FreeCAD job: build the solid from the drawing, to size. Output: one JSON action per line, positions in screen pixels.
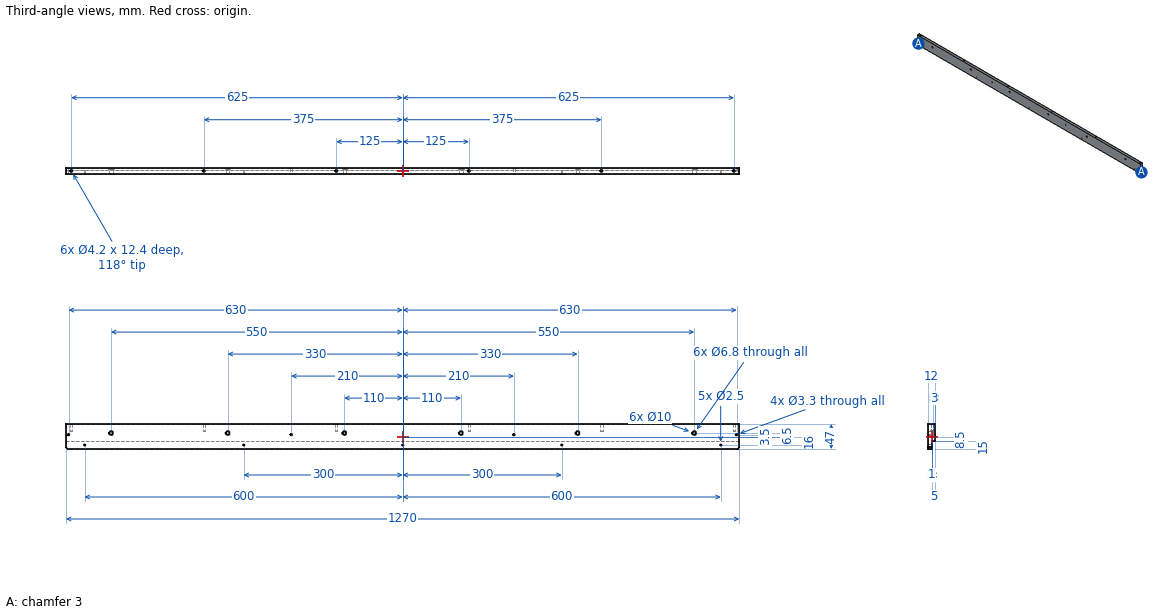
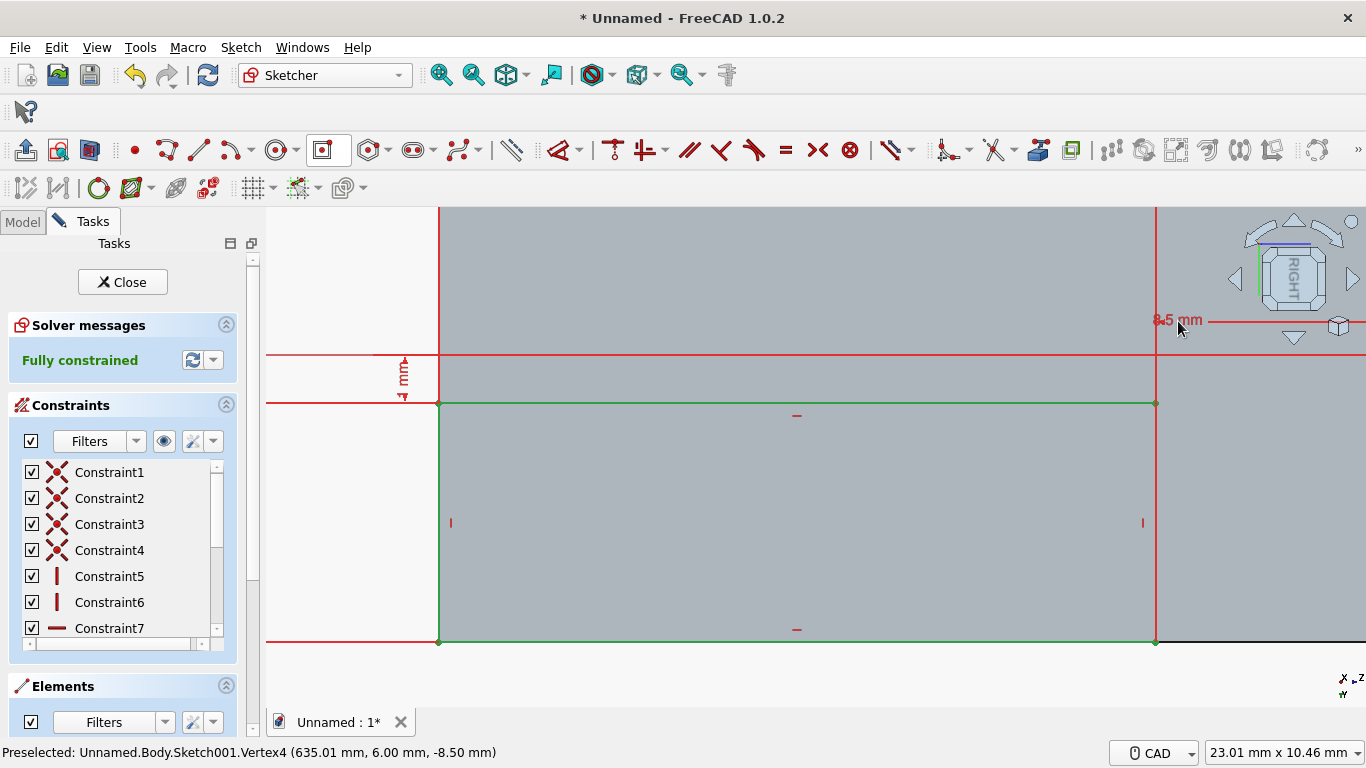
{"action": "left_click", "coordinate": [123, 282]}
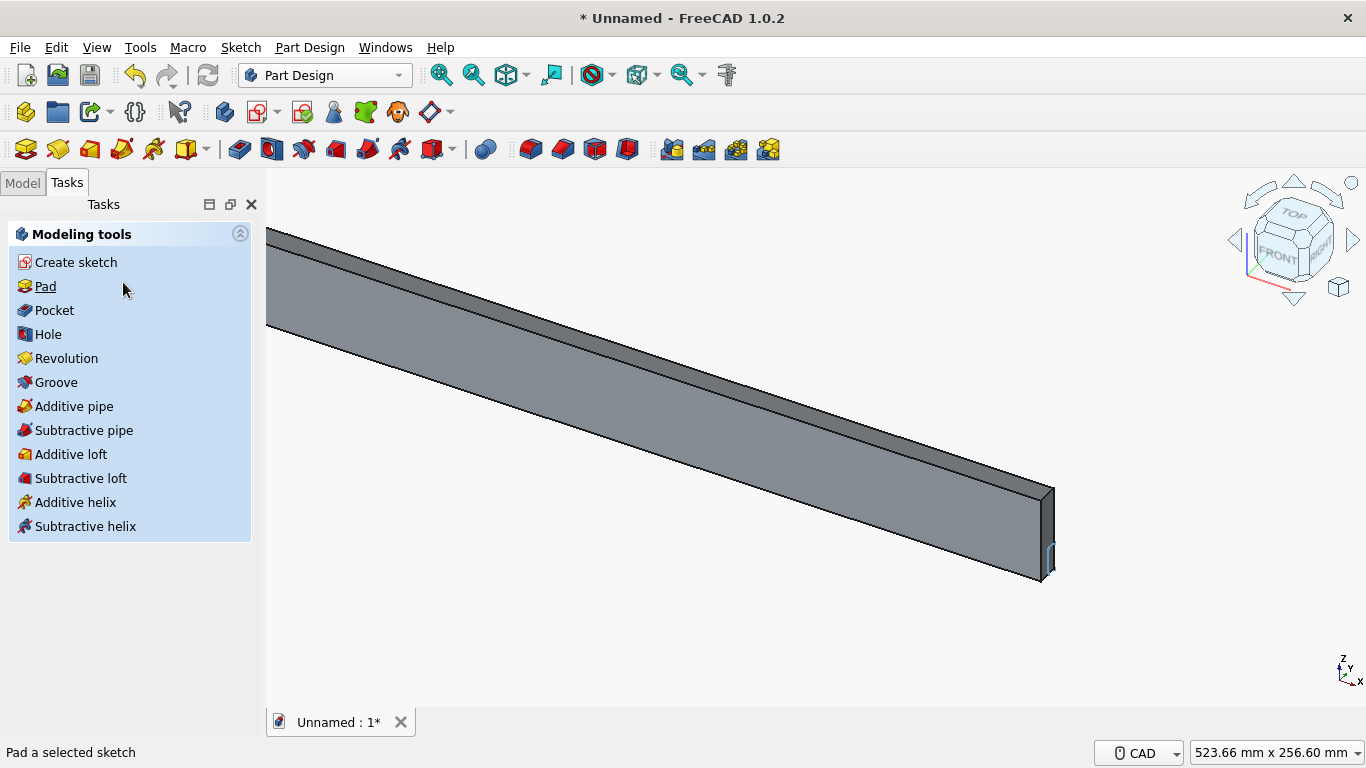
{"action": "left_click", "coordinate": [240, 150]}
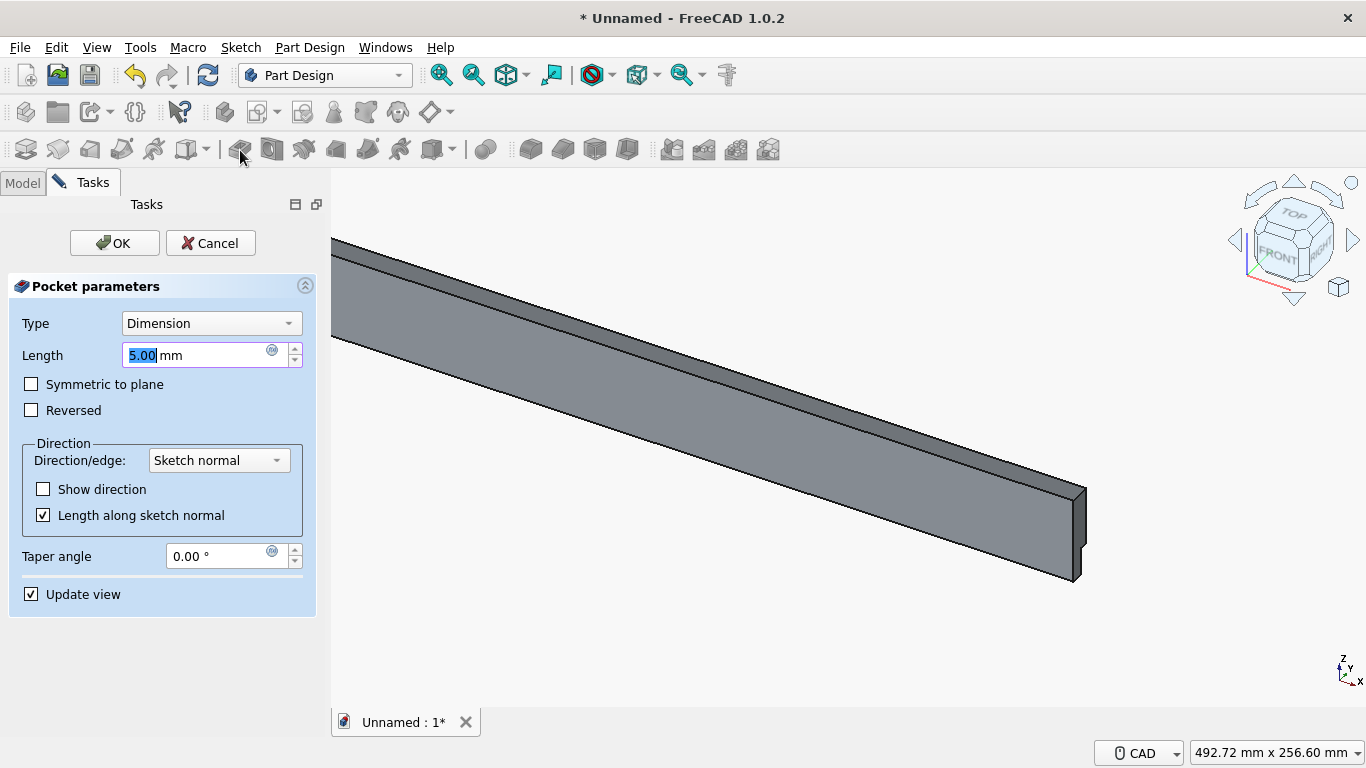
{"action": "left_click", "coordinate": [212, 324]}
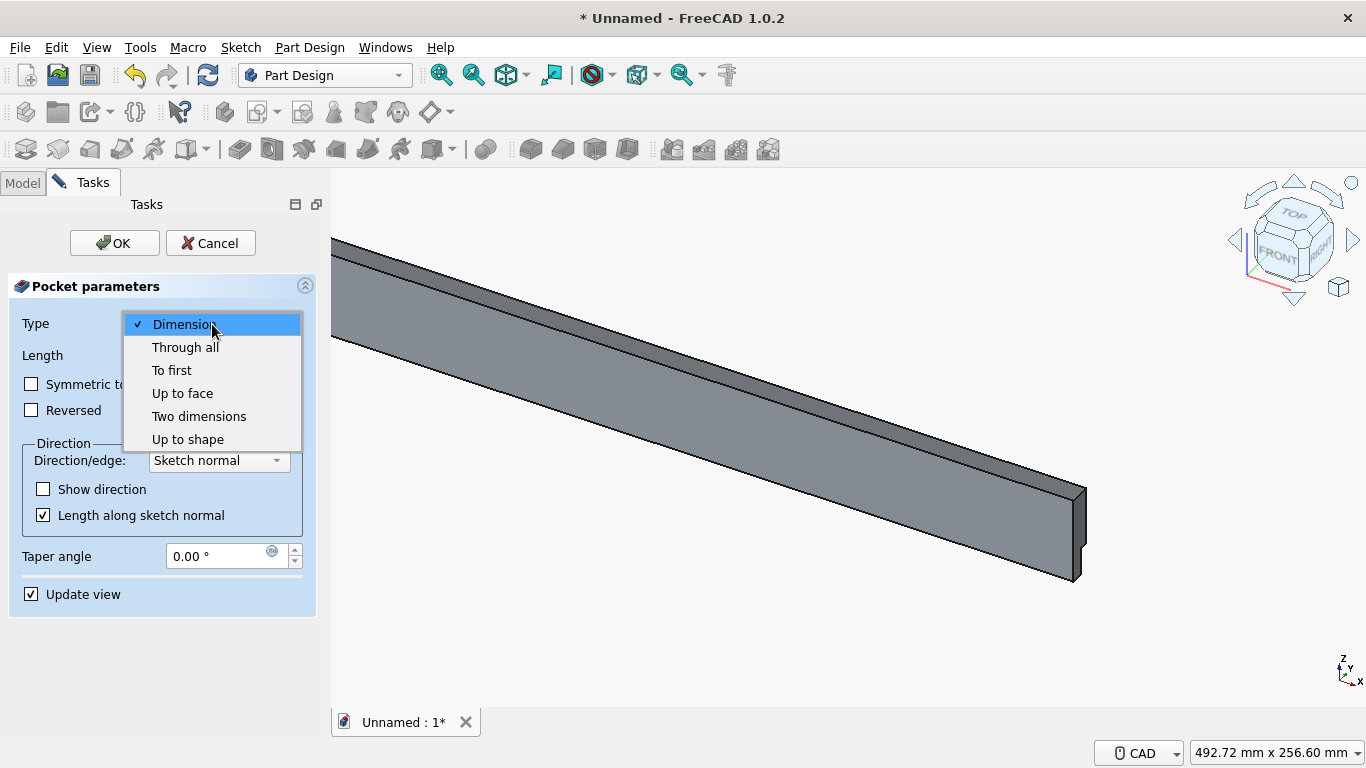
{"action": "left_click", "coordinate": [212, 348]}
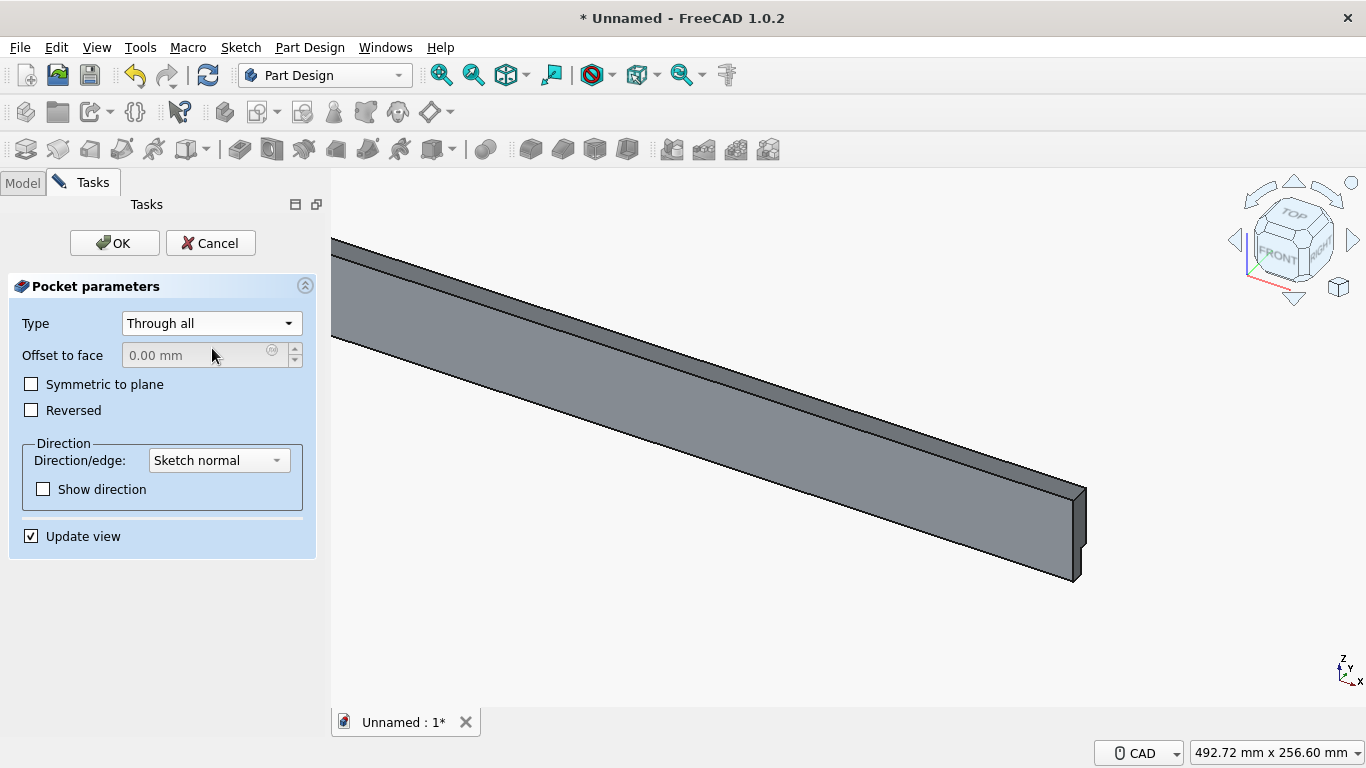
{"action": "left_click", "coordinate": [115, 243]}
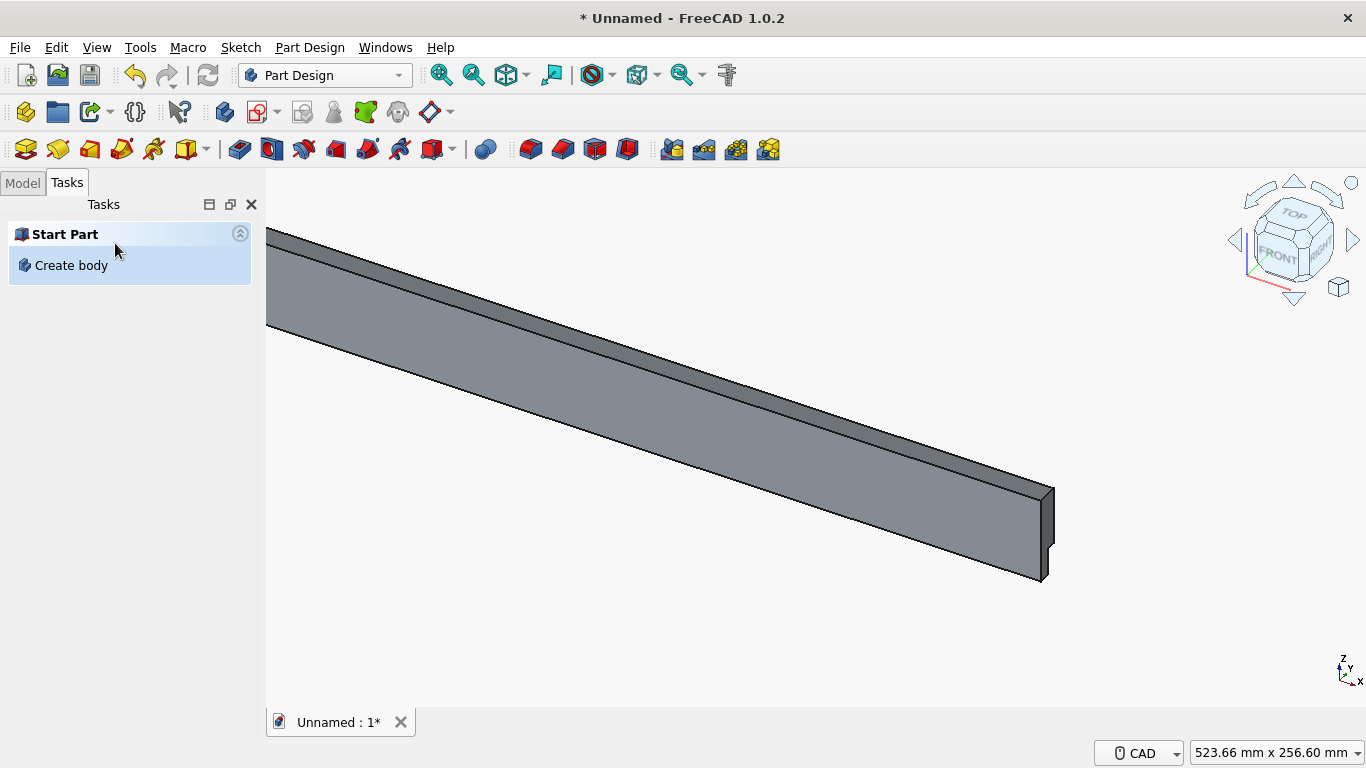
{"action": "left_click", "coordinate": [442, 76]}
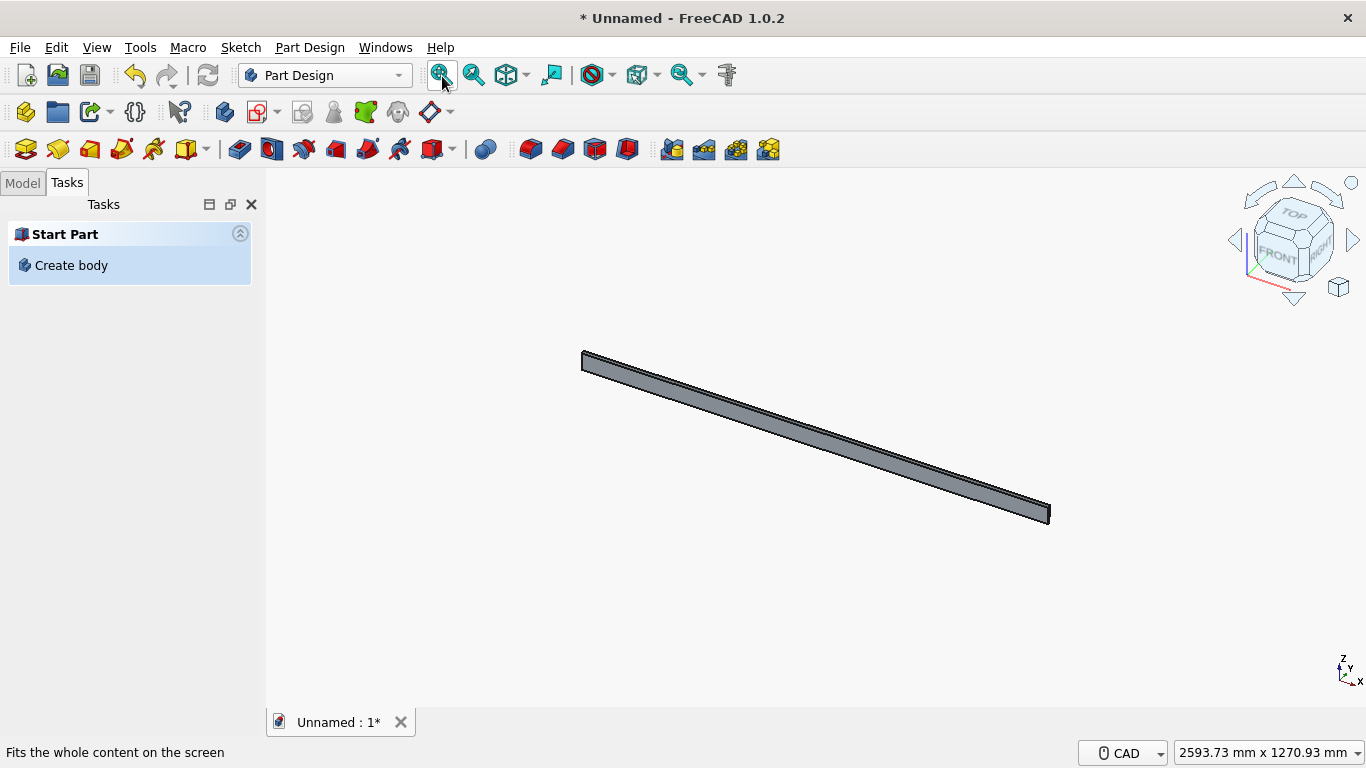
{"action": "scroll", "coordinate": [582, 368], "scroll_direction": "up", "scroll_amount": 14}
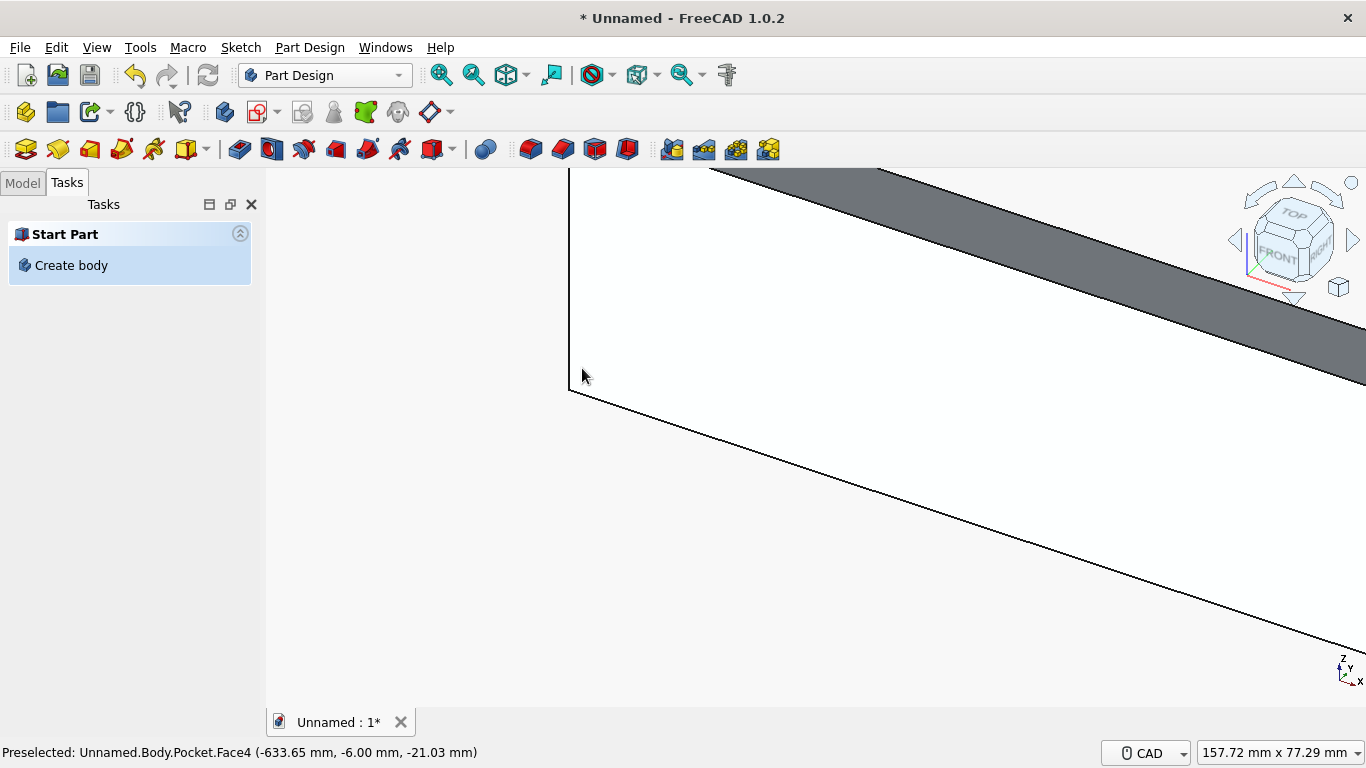
{"action": "left_click", "coordinate": [442, 76]}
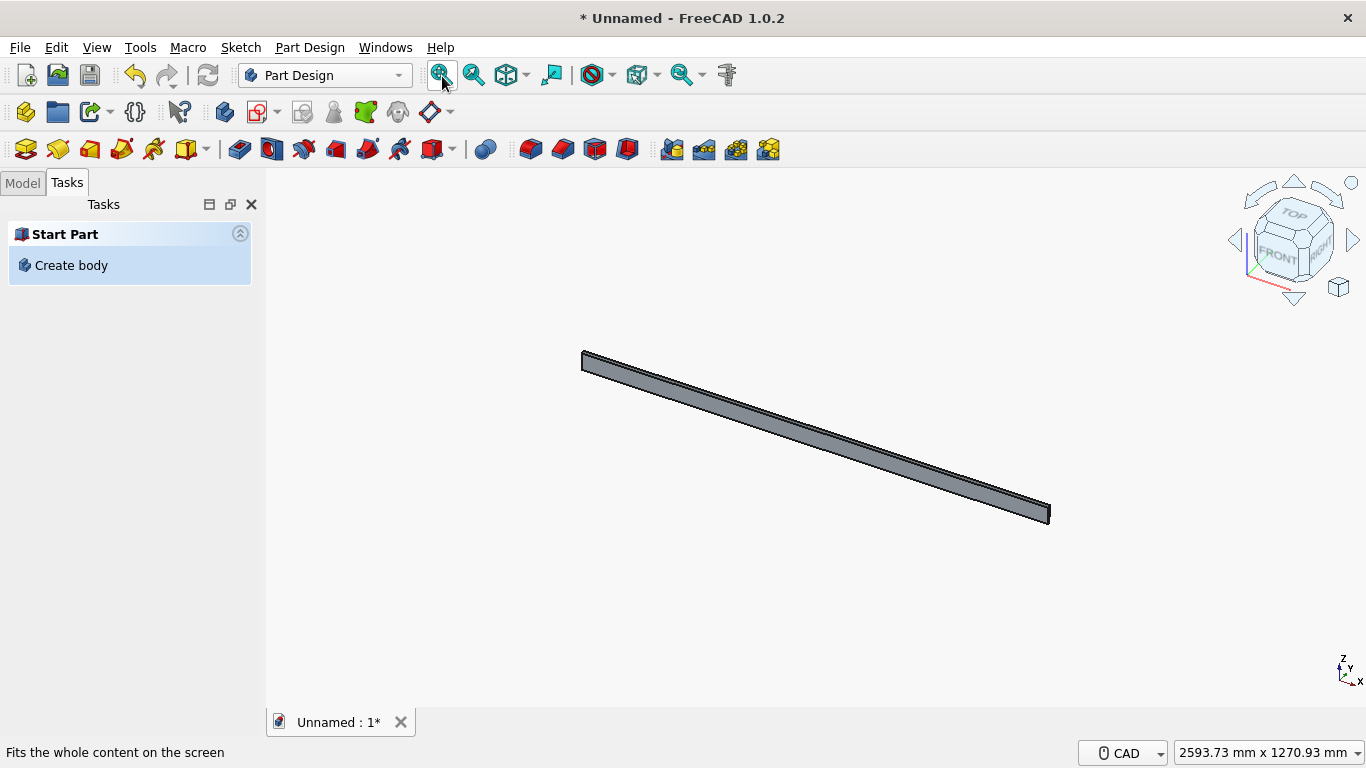
{"action": "key", "text": "0"}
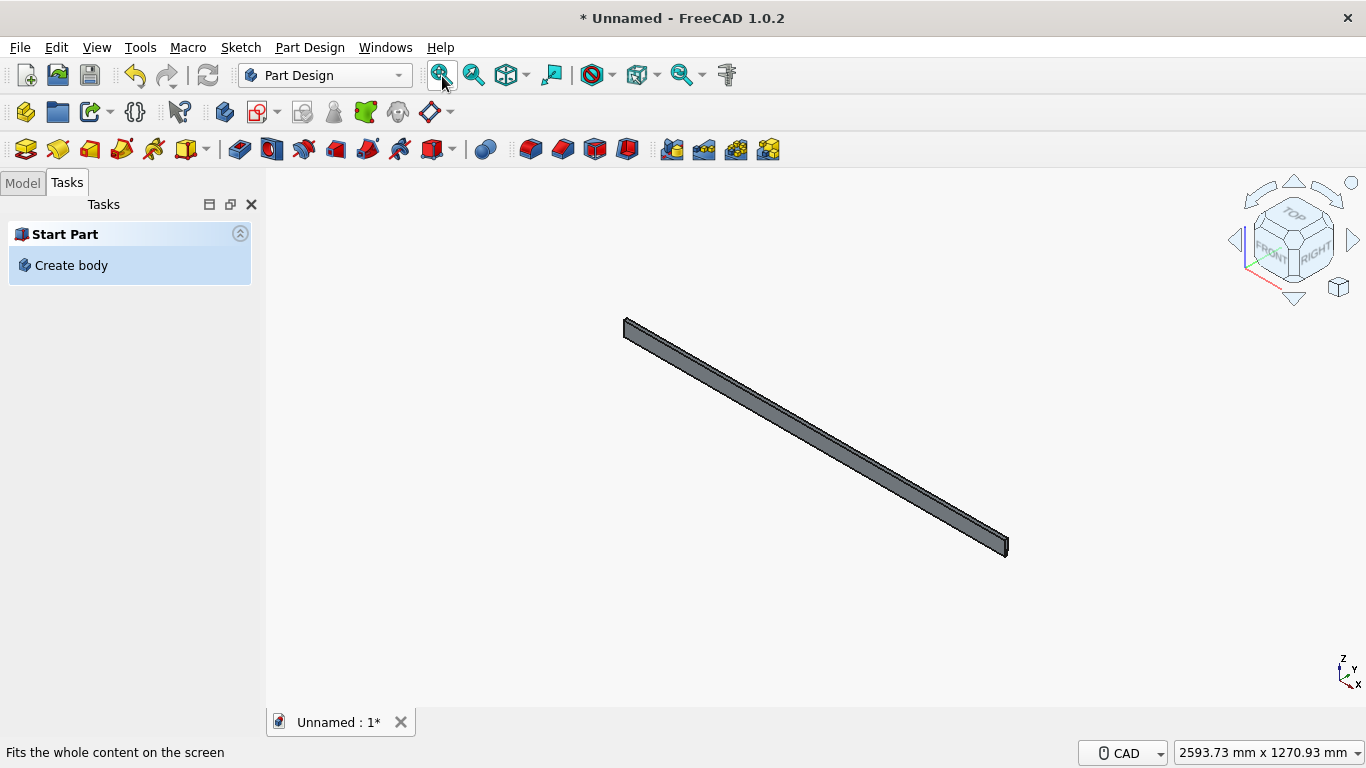
{"action": "key", "text": "v f"}